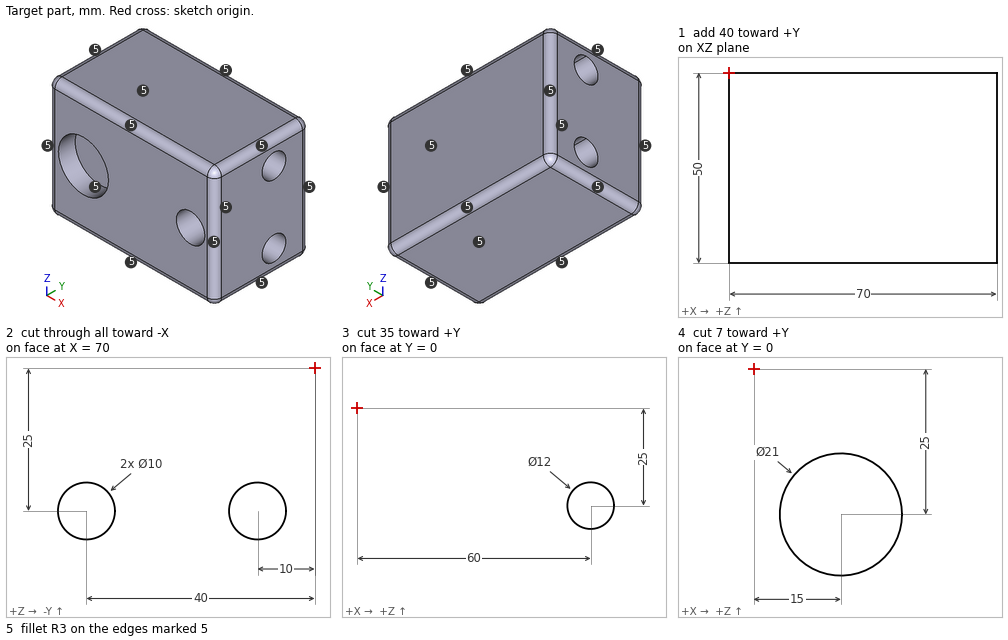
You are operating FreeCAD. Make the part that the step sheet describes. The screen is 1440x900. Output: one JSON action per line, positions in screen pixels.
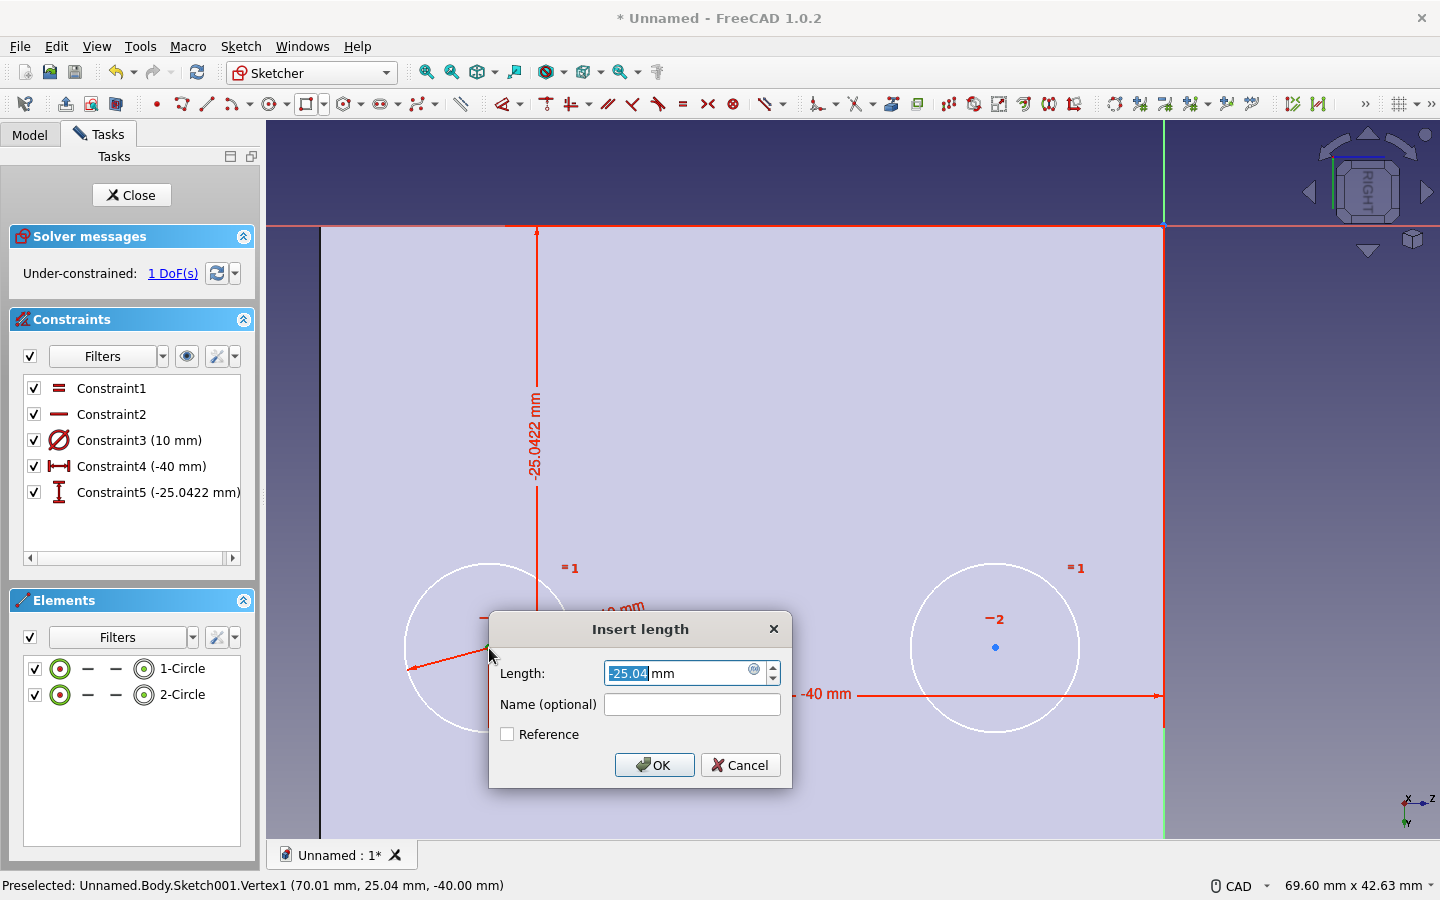
{"action": "type", "text": "-25"}
{"action": "key", "text": "Return"}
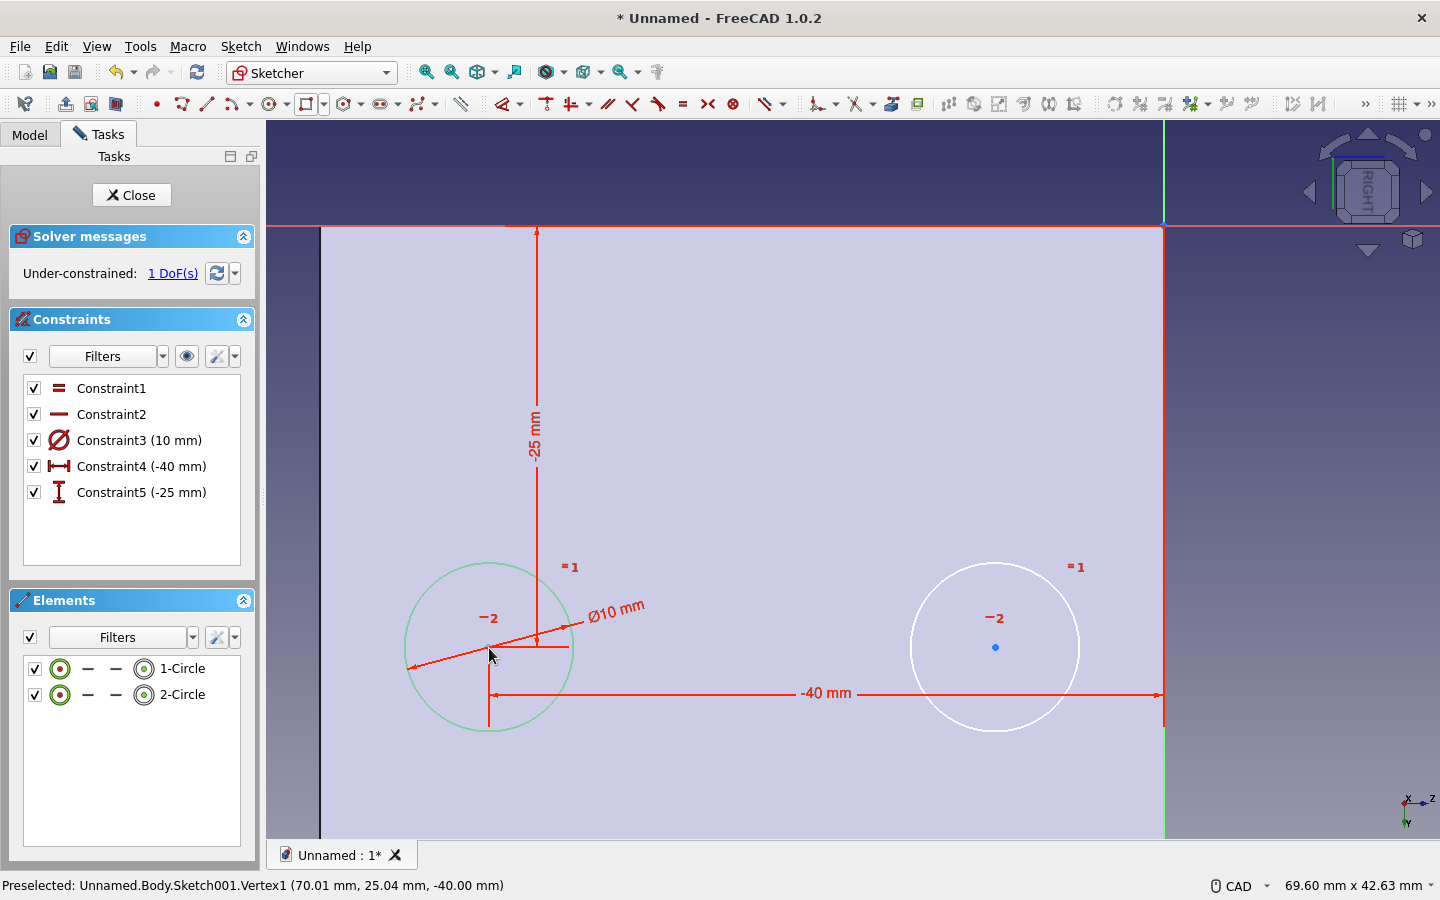
{"action": "left_click", "coordinate": [995, 647]}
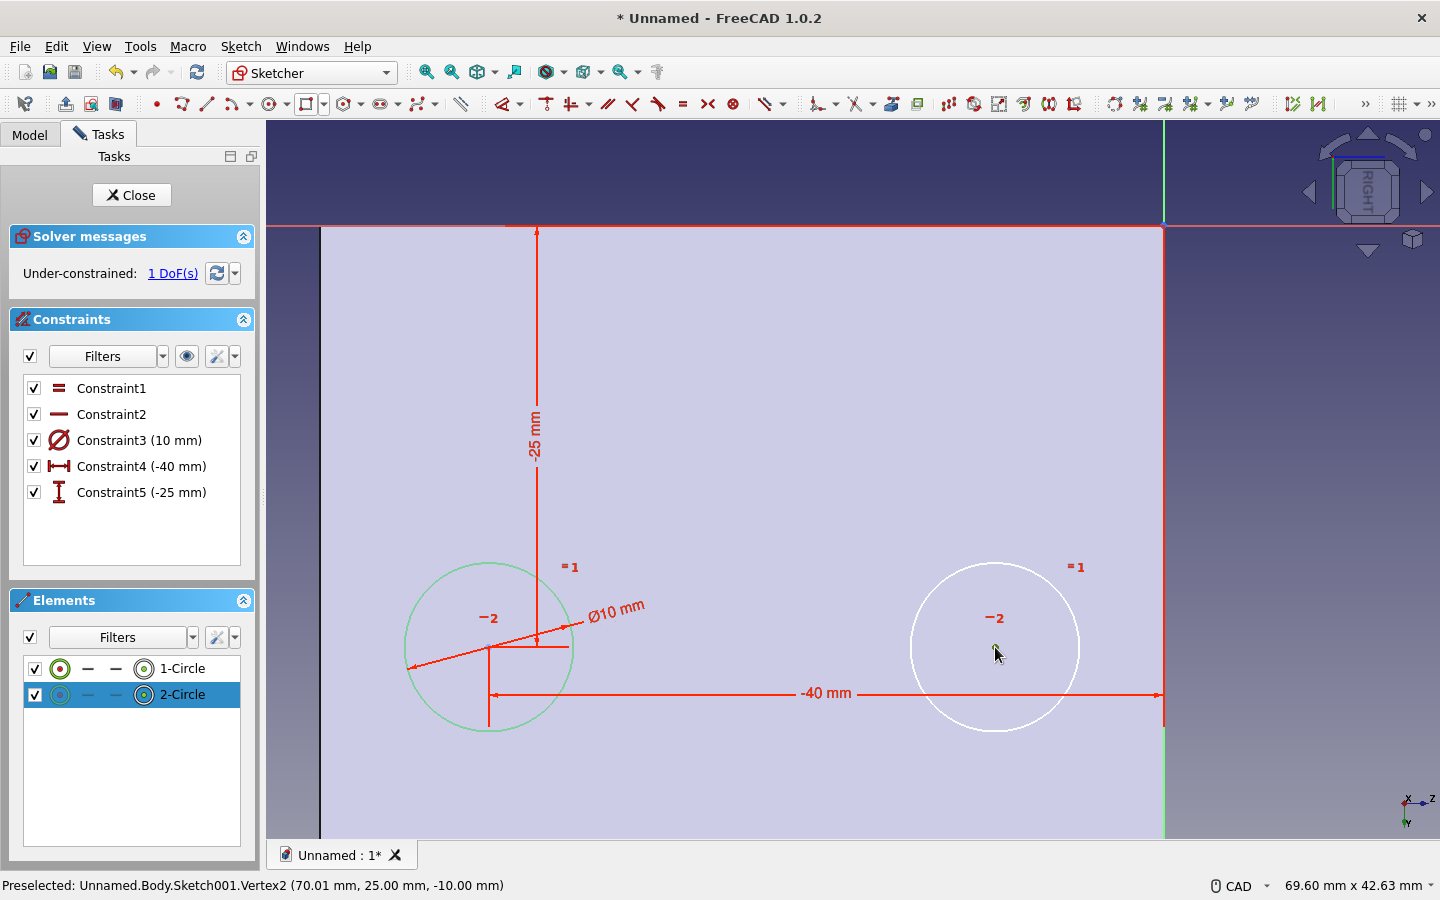
{"action": "key", "text": "l"}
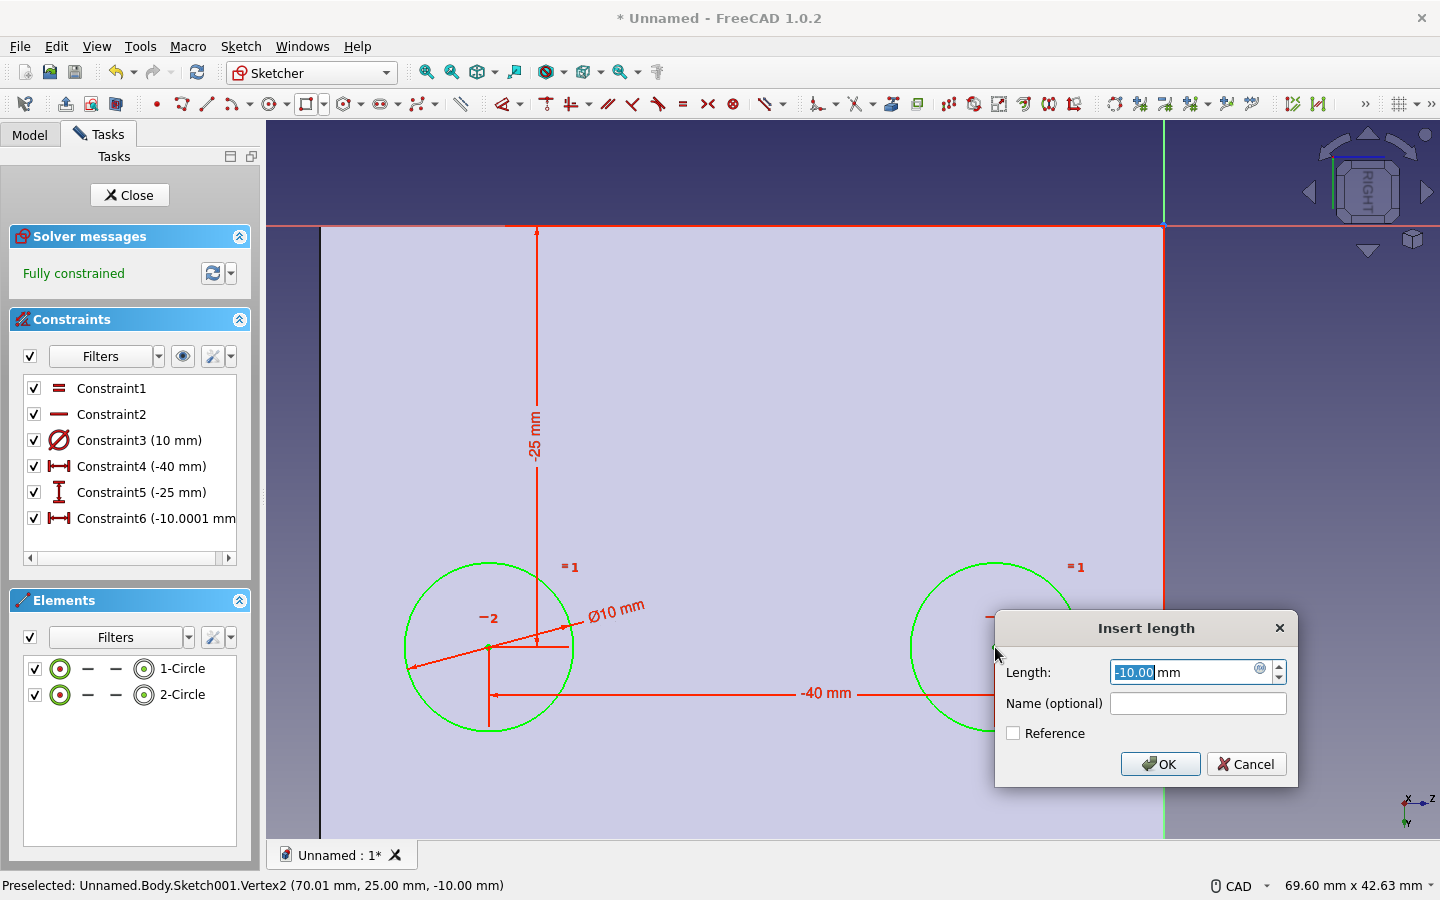
{"action": "type", "text": "-10"}
{"action": "key", "text": "Return"}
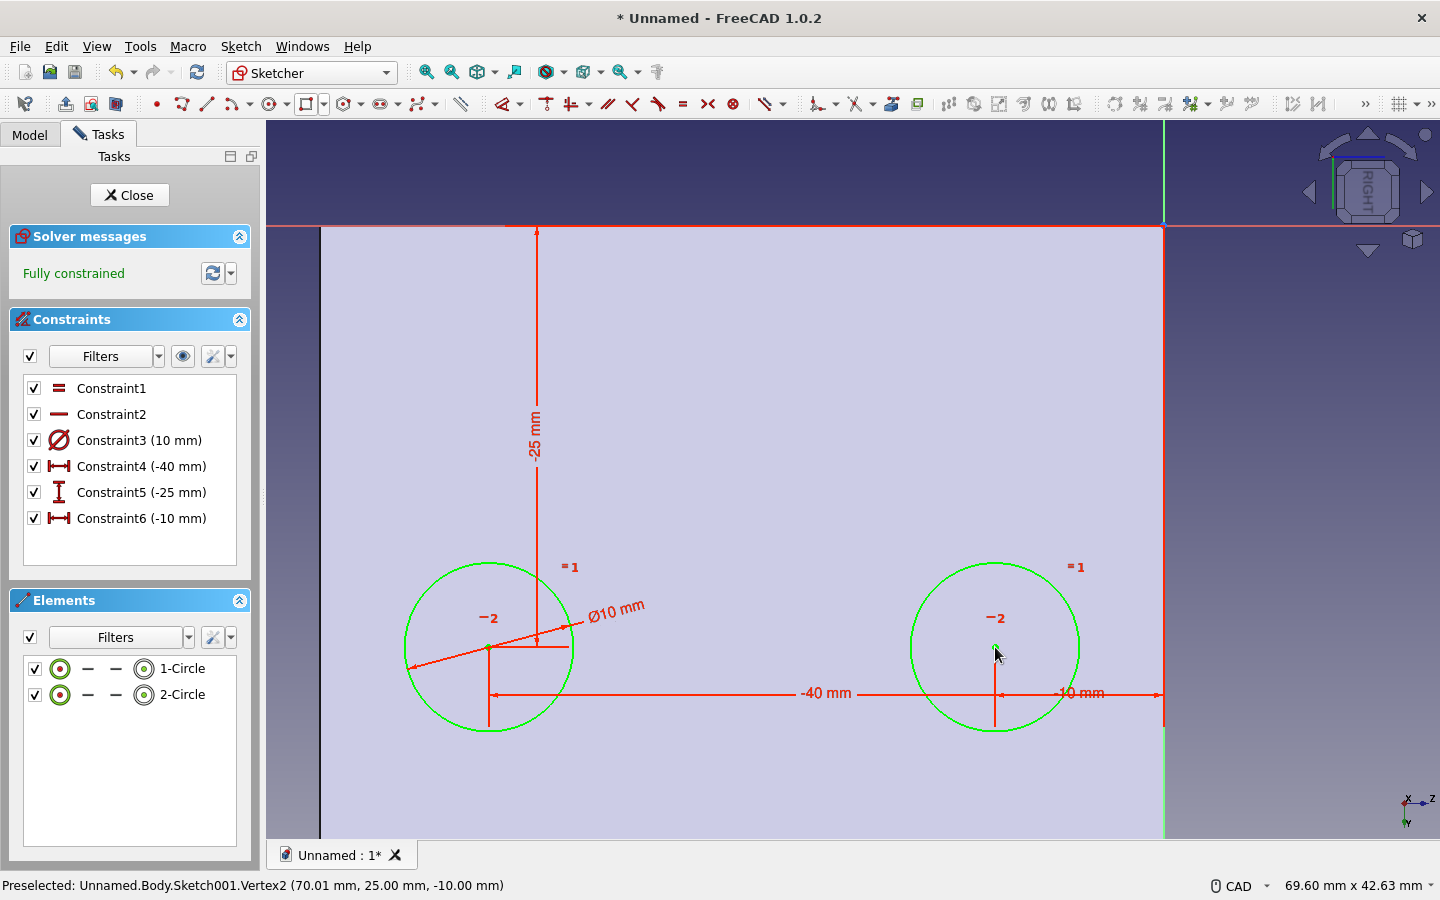
{"action": "left_click", "coordinate": [130, 195]}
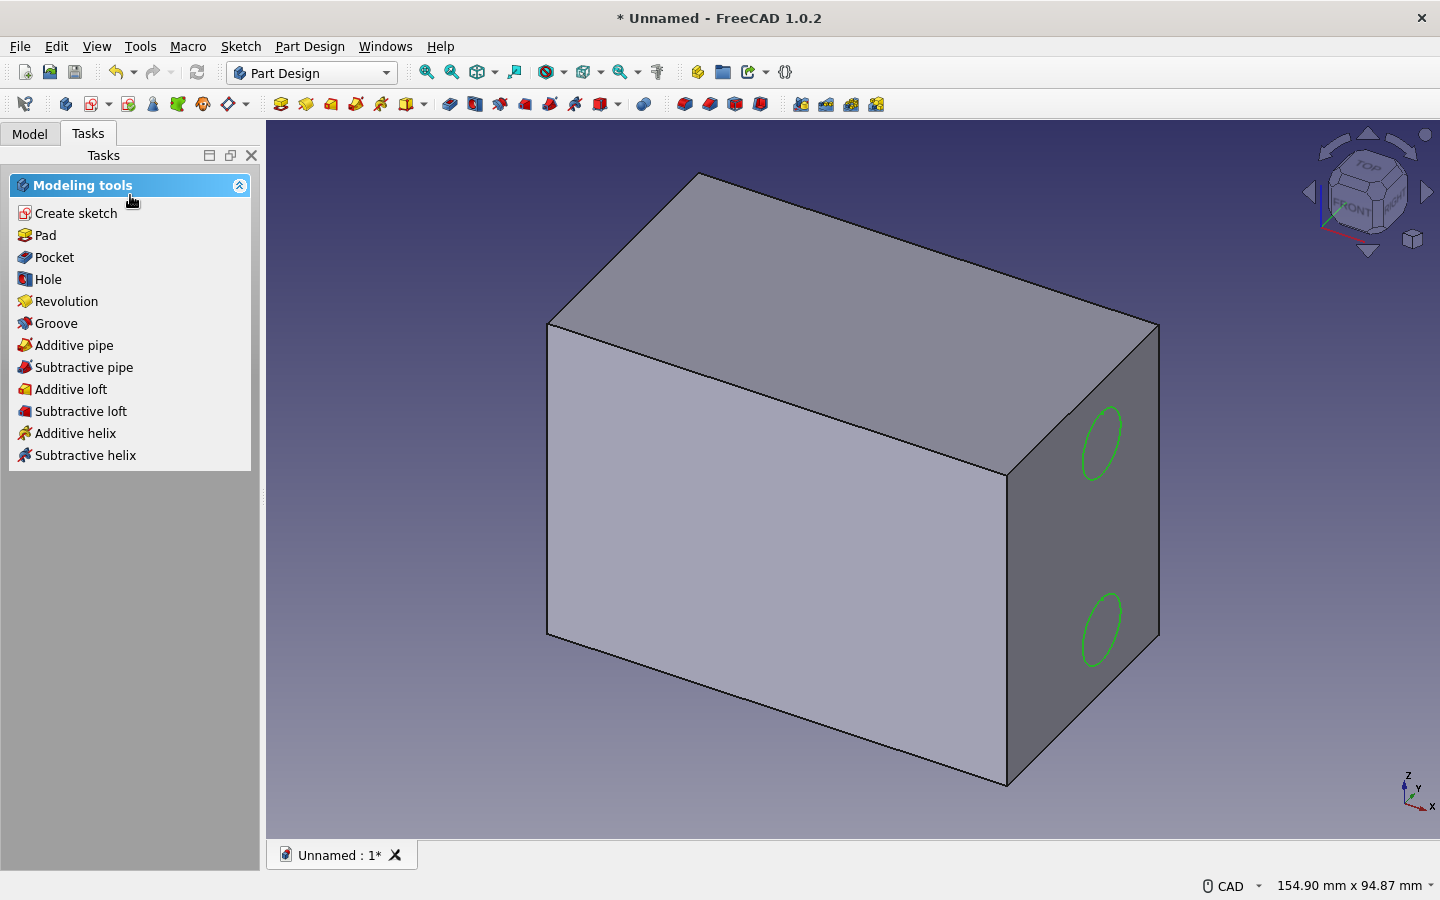
{"action": "left_click", "coordinate": [450, 104]}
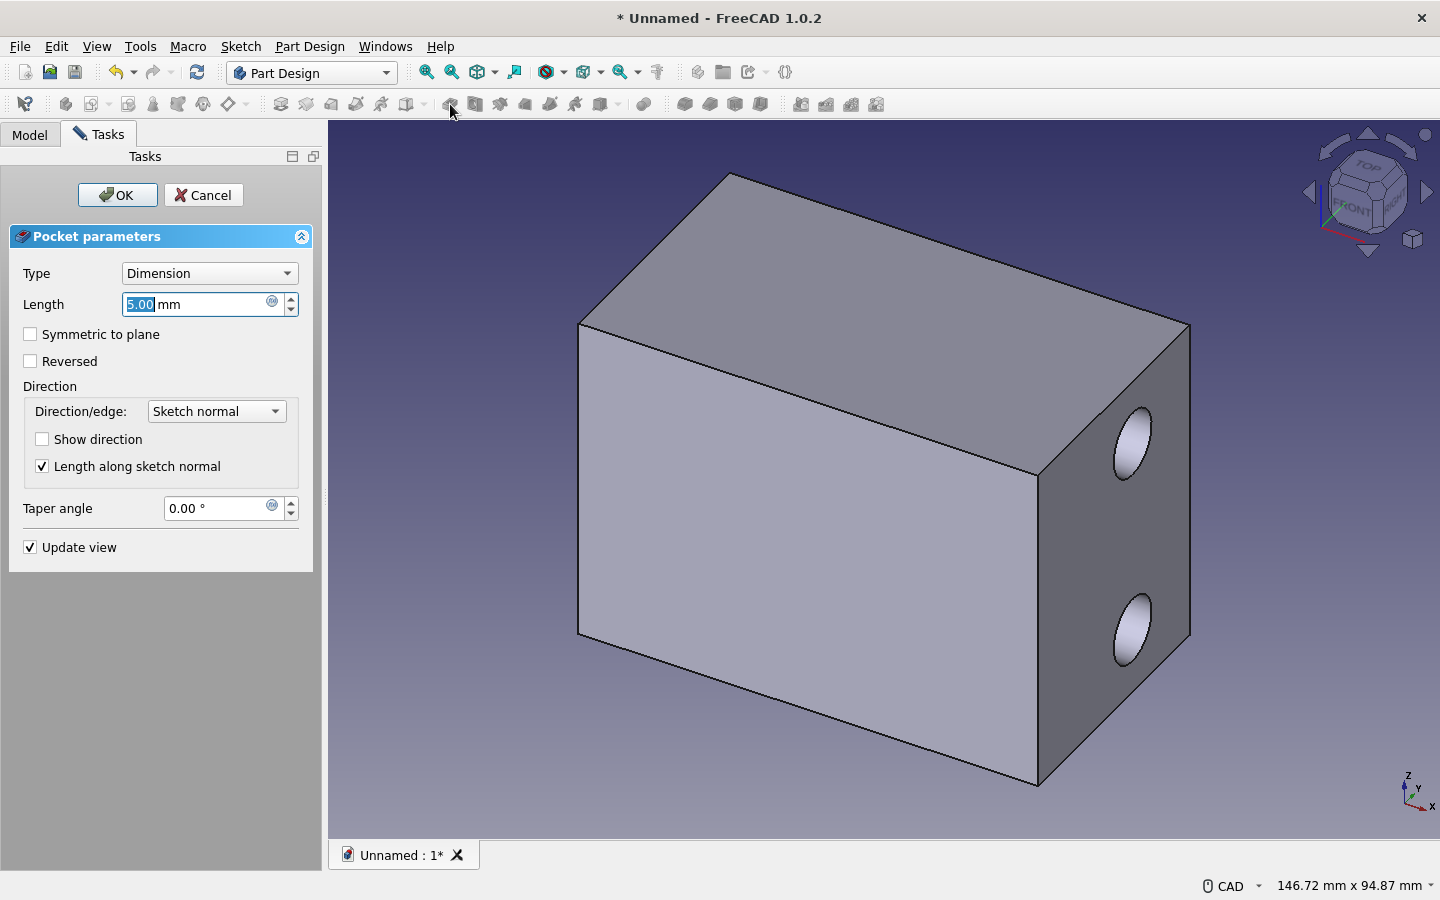
{"action": "left_click", "coordinate": [210, 274]}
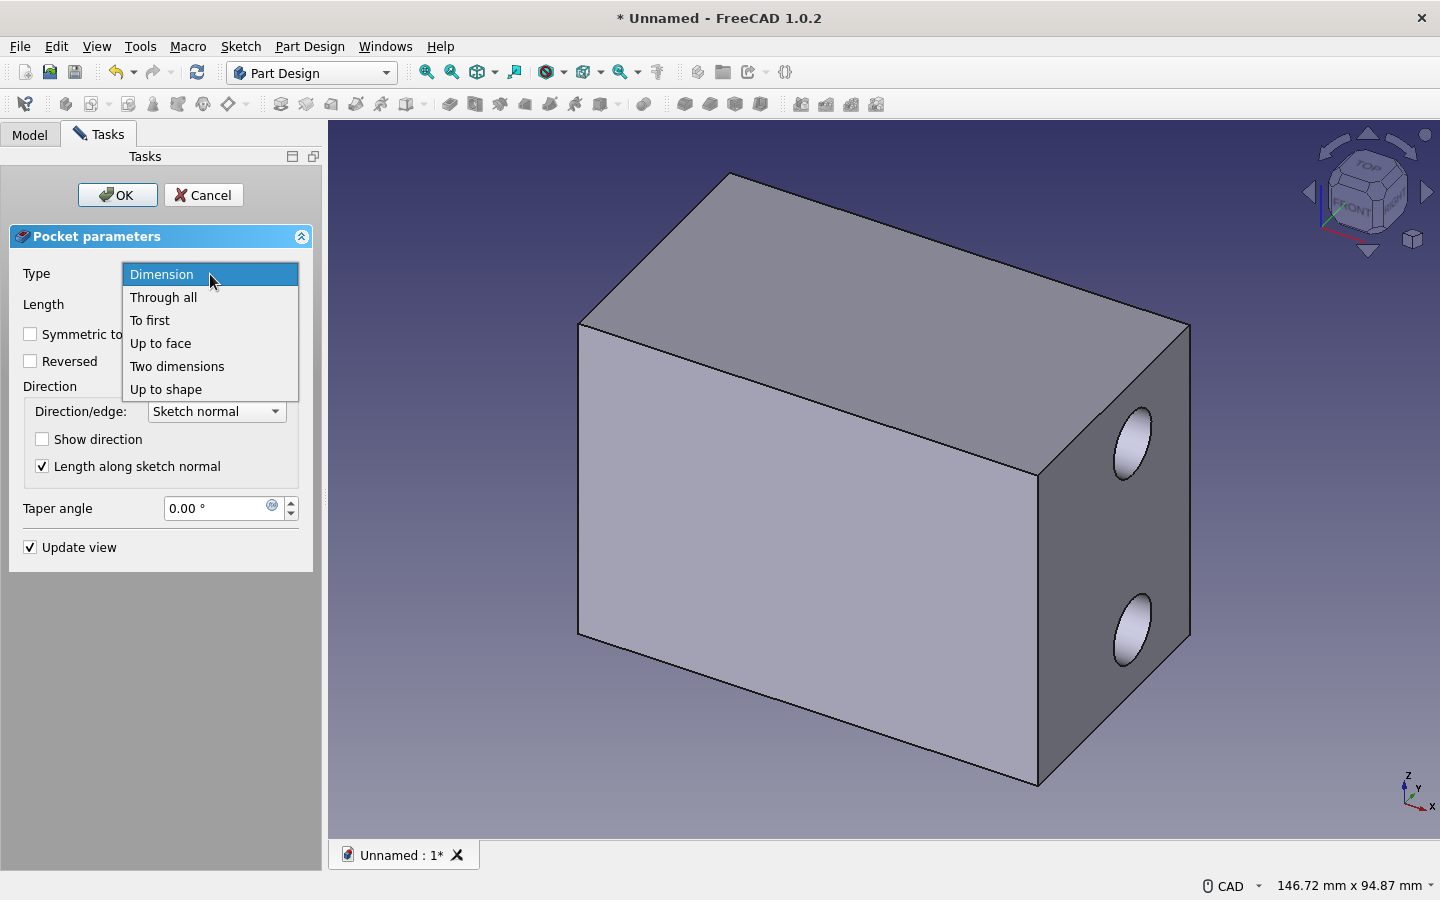
{"action": "left_click", "coordinate": [208, 298]}